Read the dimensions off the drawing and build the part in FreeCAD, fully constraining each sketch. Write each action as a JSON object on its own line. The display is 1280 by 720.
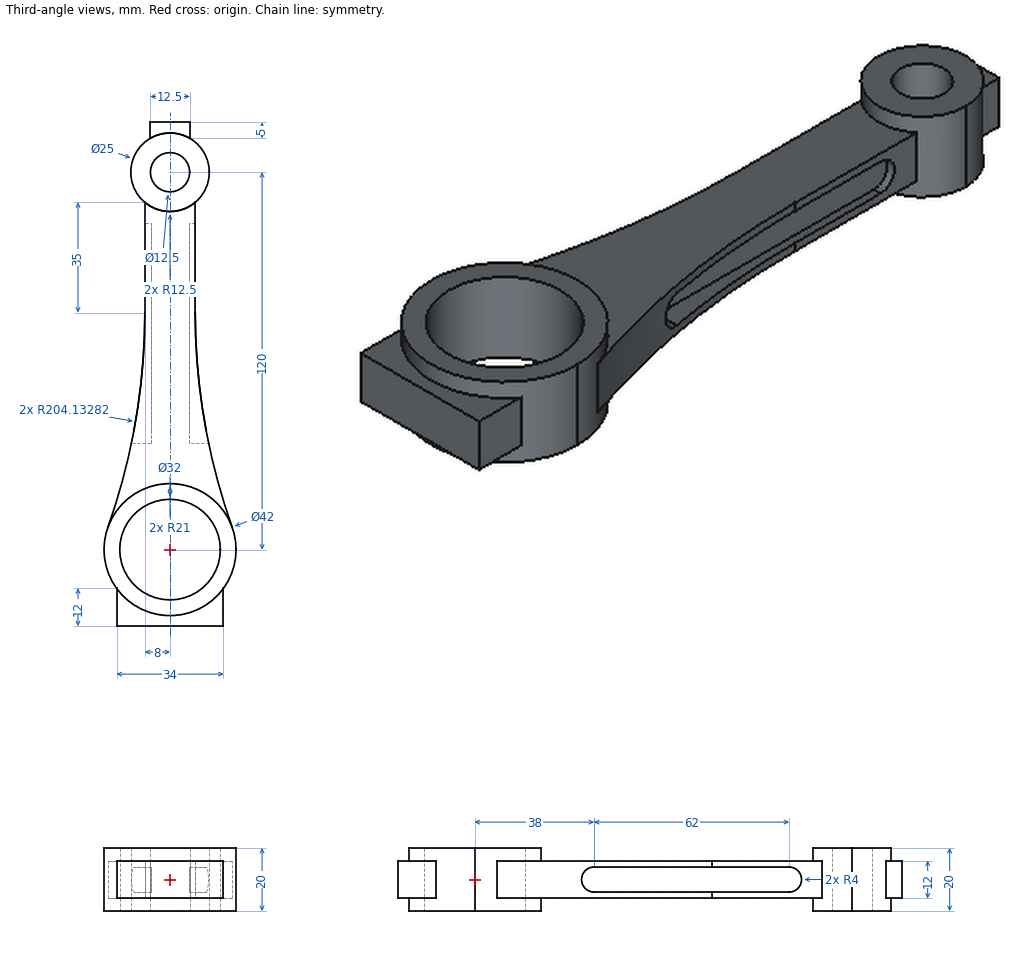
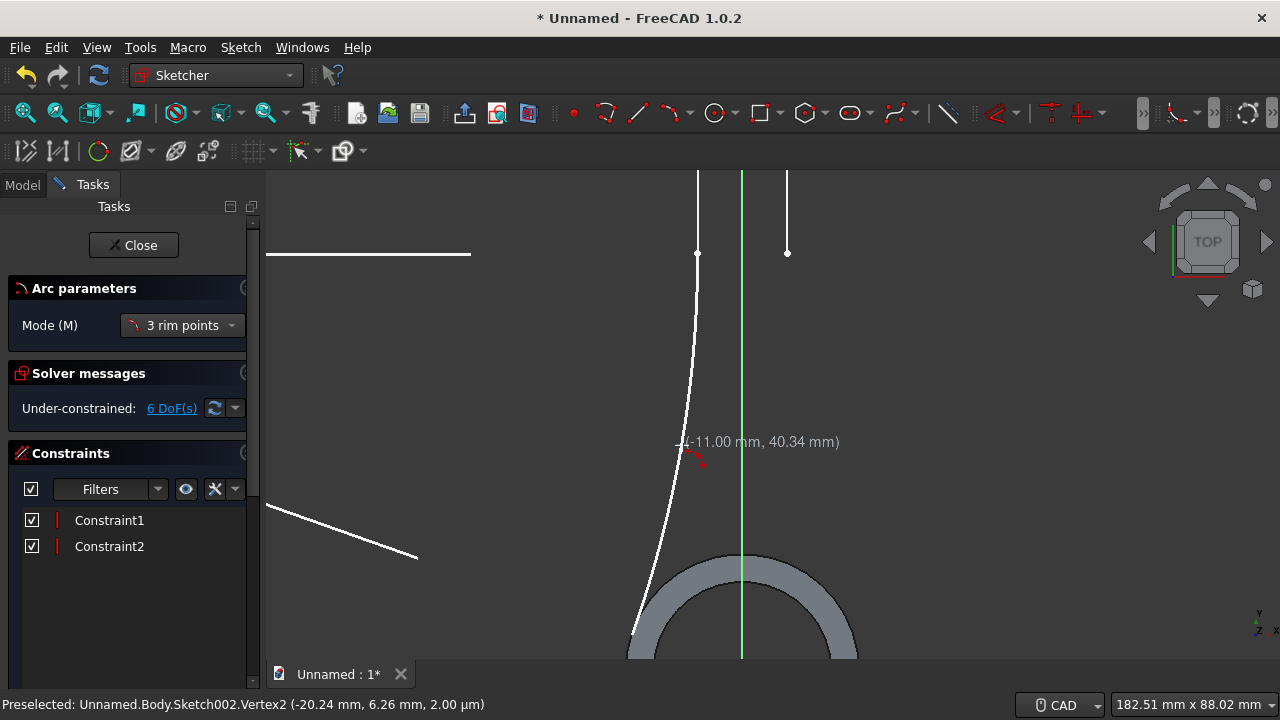
{"action": "left_click", "coordinate": [681, 445]}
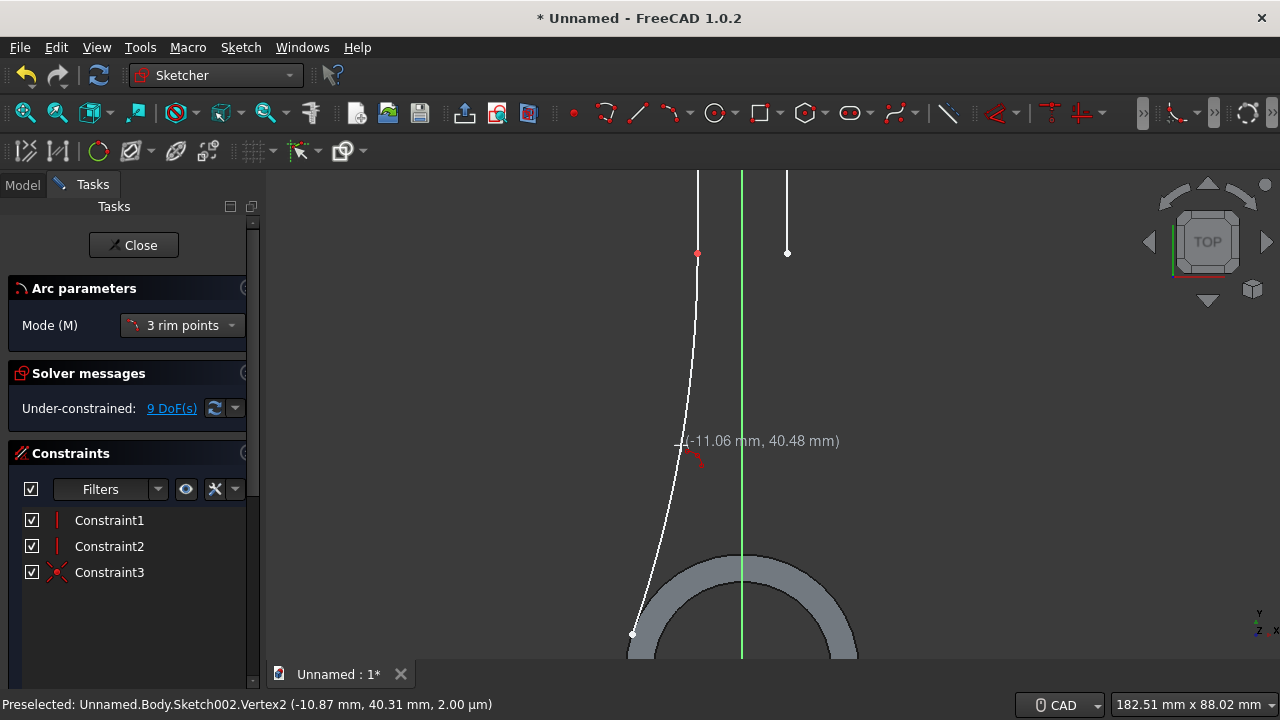
{"action": "scroll", "coordinate": [682, 446], "scroll_direction": "down", "scroll_amount": 5}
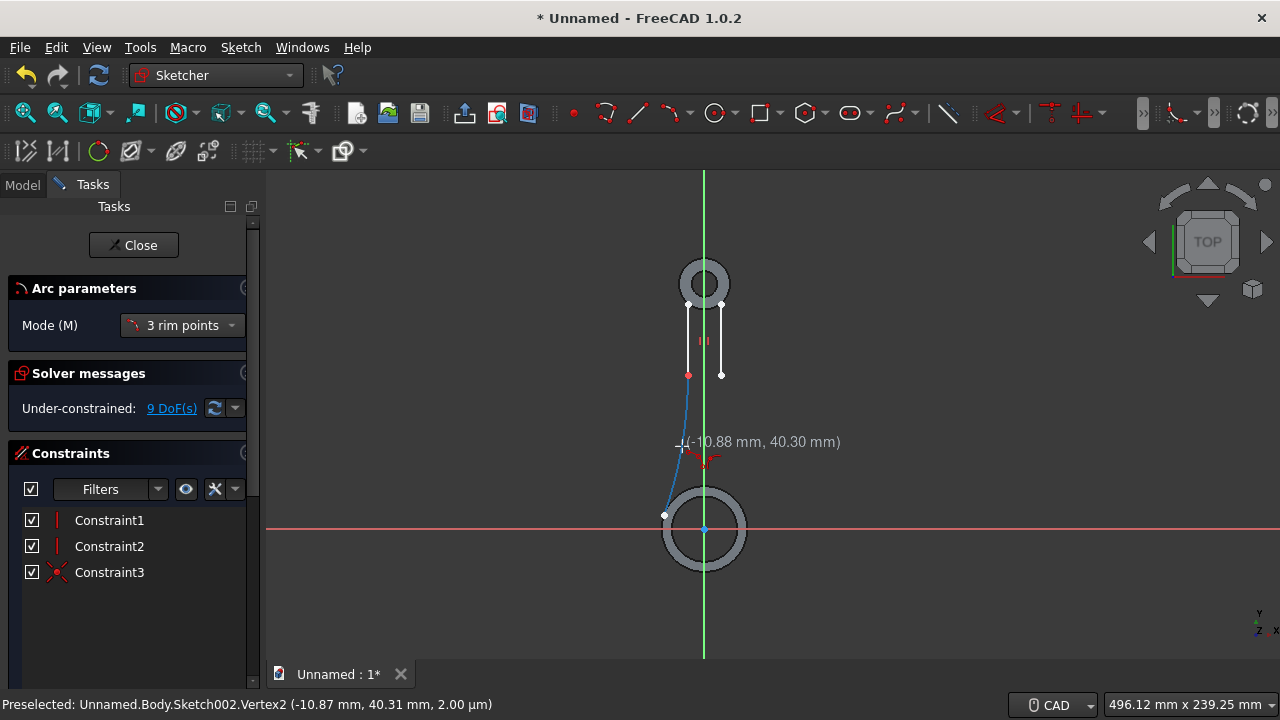
{"action": "left_click", "coordinate": [664, 516]}
{"action": "left_click", "coordinate": [745, 515]}
{"action": "left_click", "coordinate": [725, 491]}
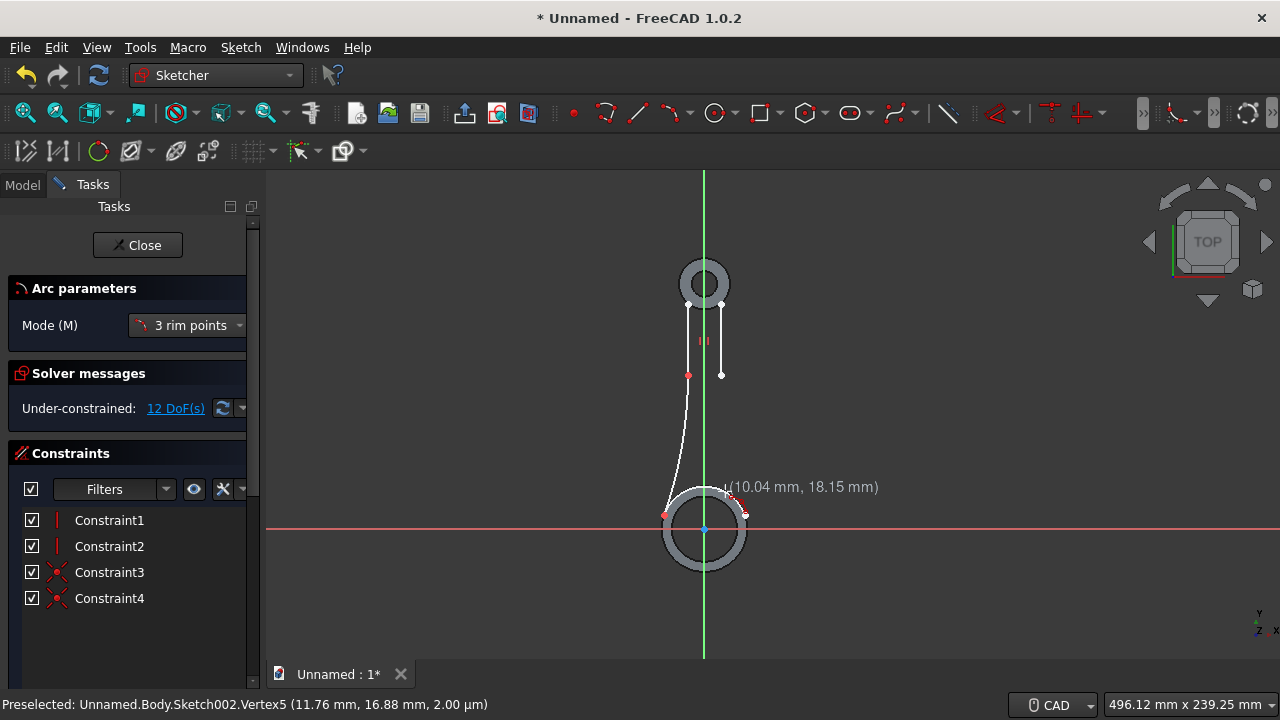
{"action": "left_click", "coordinate": [745, 516]}
{"action": "left_click", "coordinate": [721, 376]}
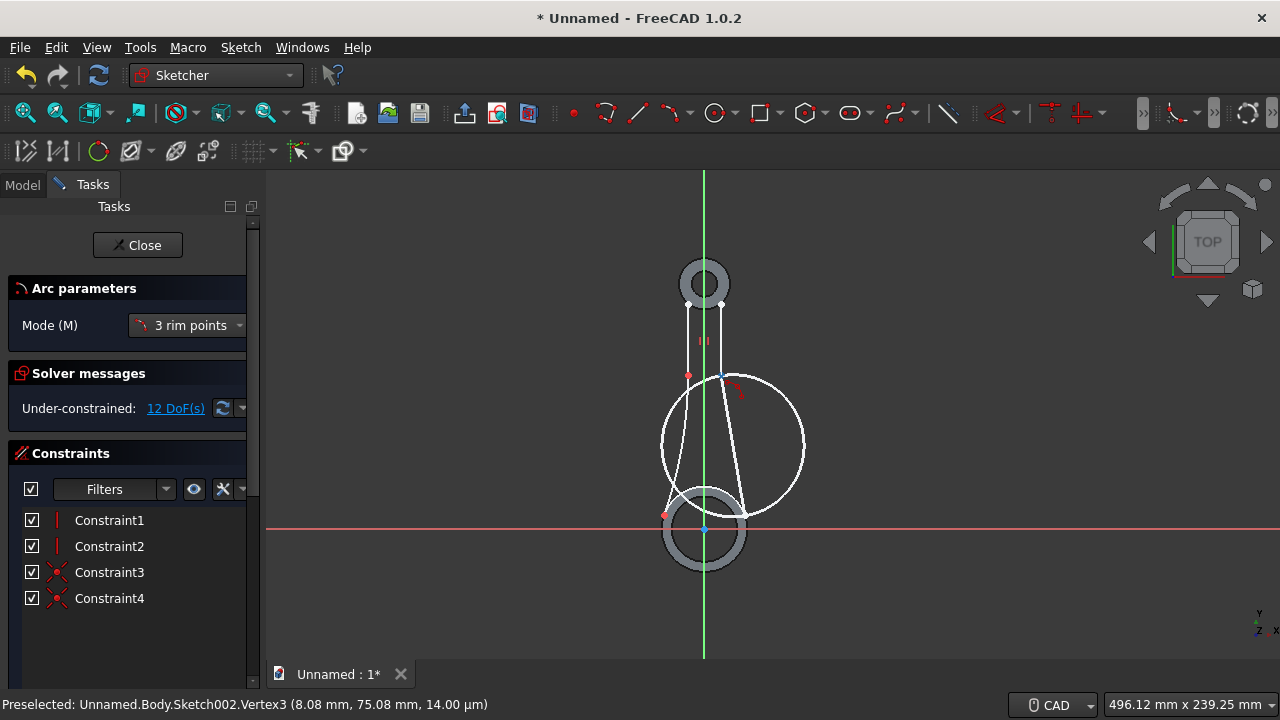
{"action": "scroll", "coordinate": [727, 446], "scroll_direction": "up", "scroll_amount": 5}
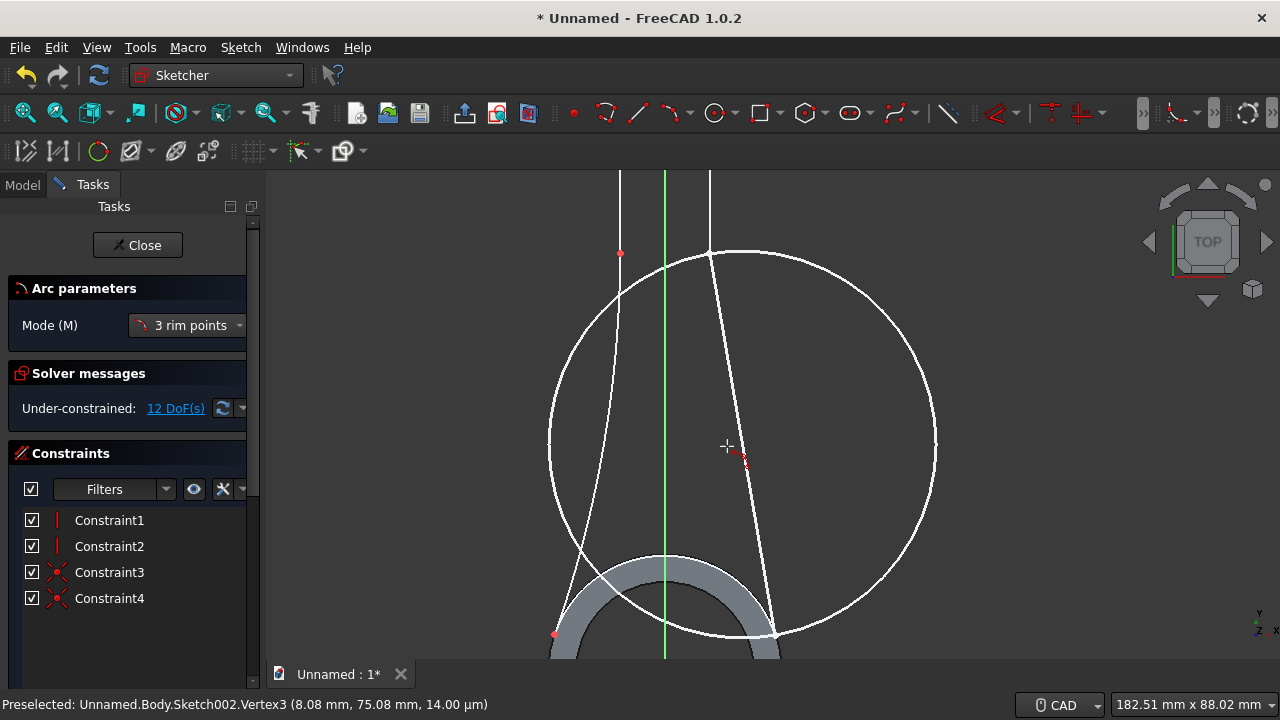
{"action": "left_click", "coordinate": [726, 445]}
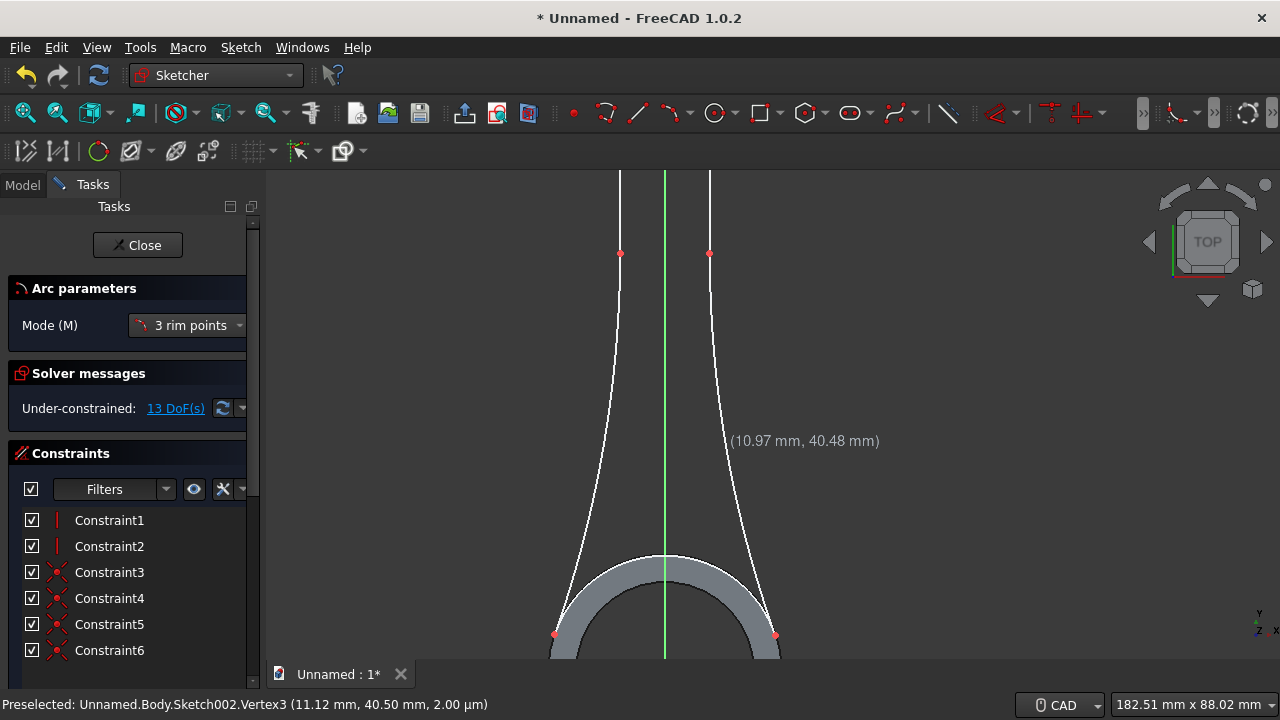
{"action": "scroll", "coordinate": [727, 446], "scroll_direction": "down", "scroll_amount": 5}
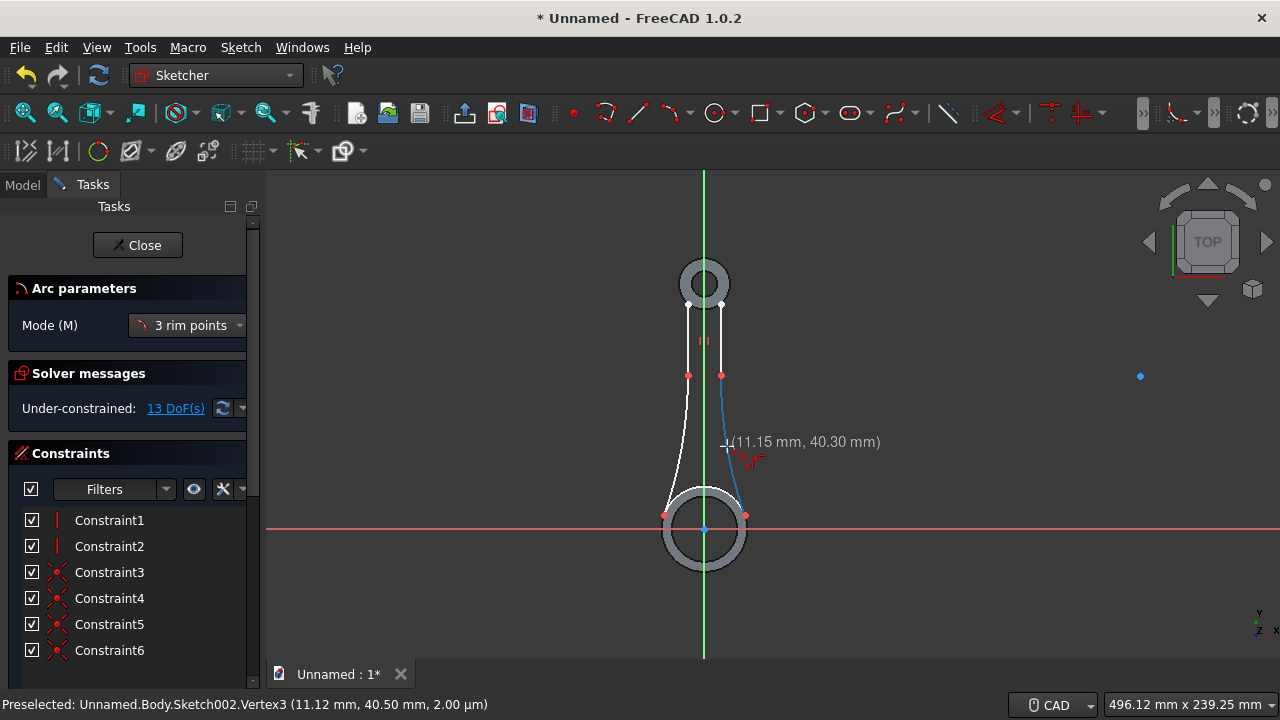
{"action": "left_click", "coordinate": [721, 305]}
{"action": "left_click", "coordinate": [688, 305]}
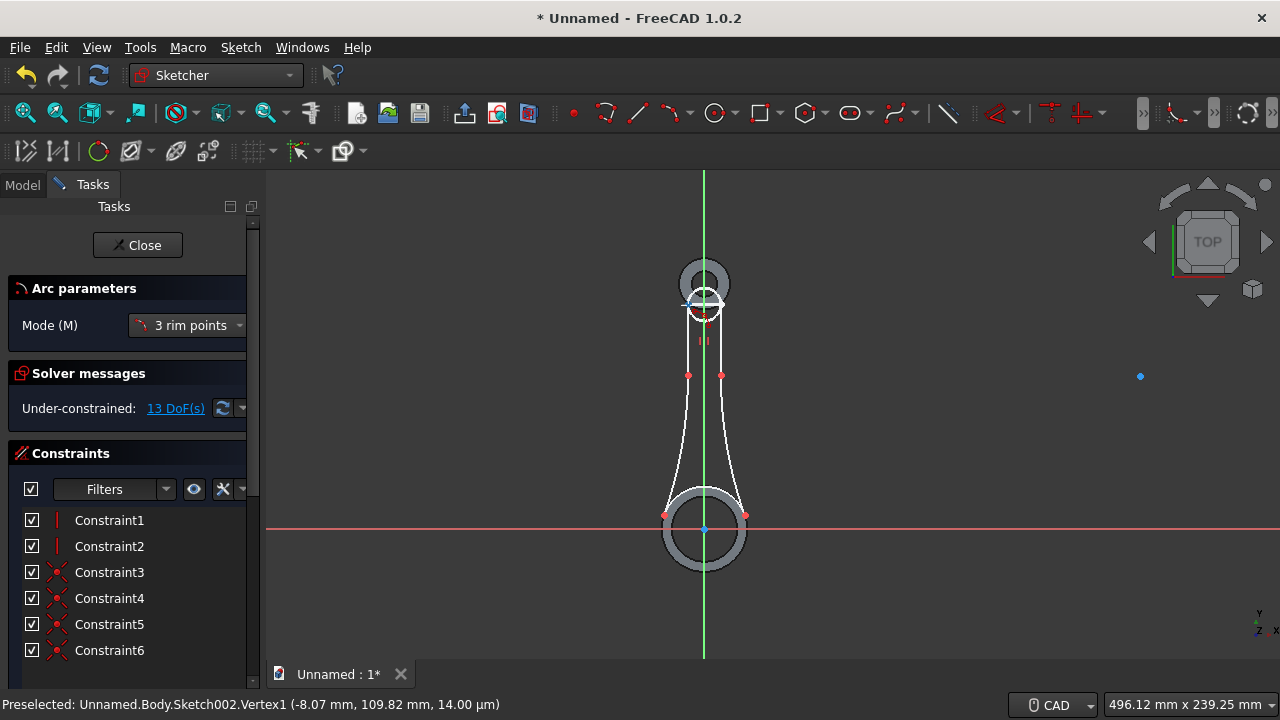
{"action": "scroll", "coordinate": [697, 308], "scroll_direction": "up", "scroll_amount": 6}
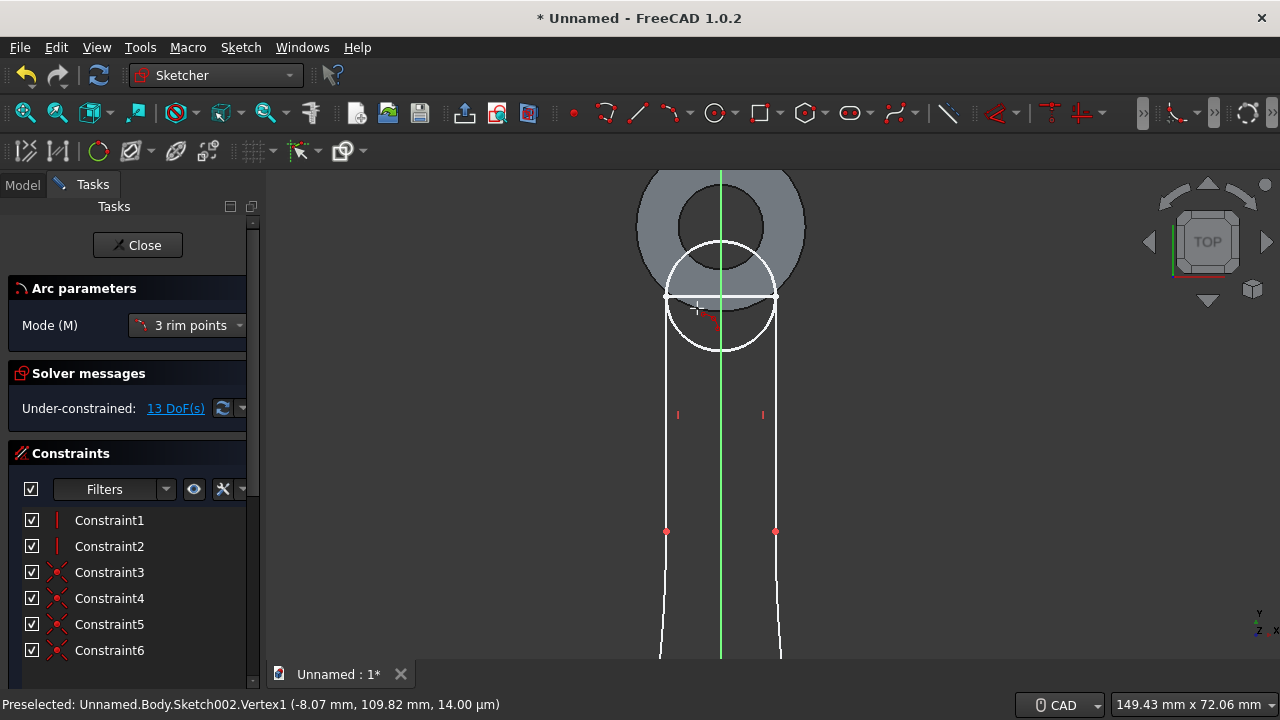
{"action": "left_click", "coordinate": [698, 309]}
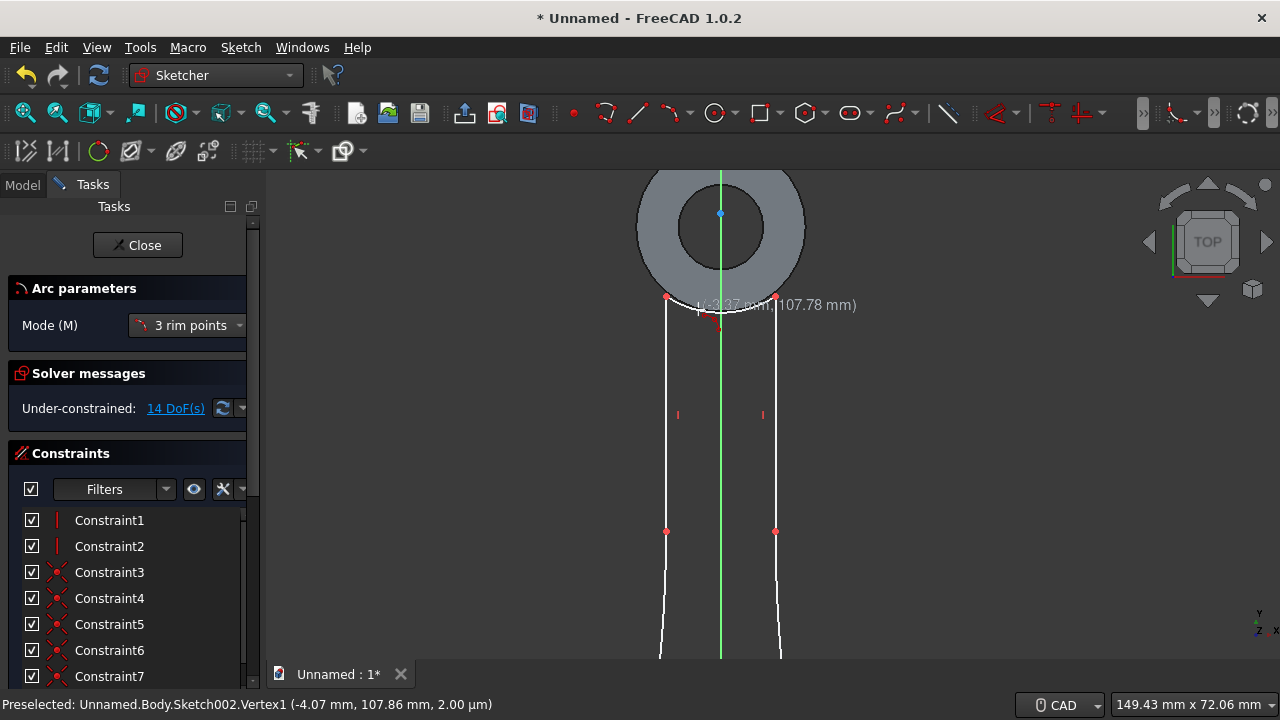
{"action": "key", "text": "g m"}